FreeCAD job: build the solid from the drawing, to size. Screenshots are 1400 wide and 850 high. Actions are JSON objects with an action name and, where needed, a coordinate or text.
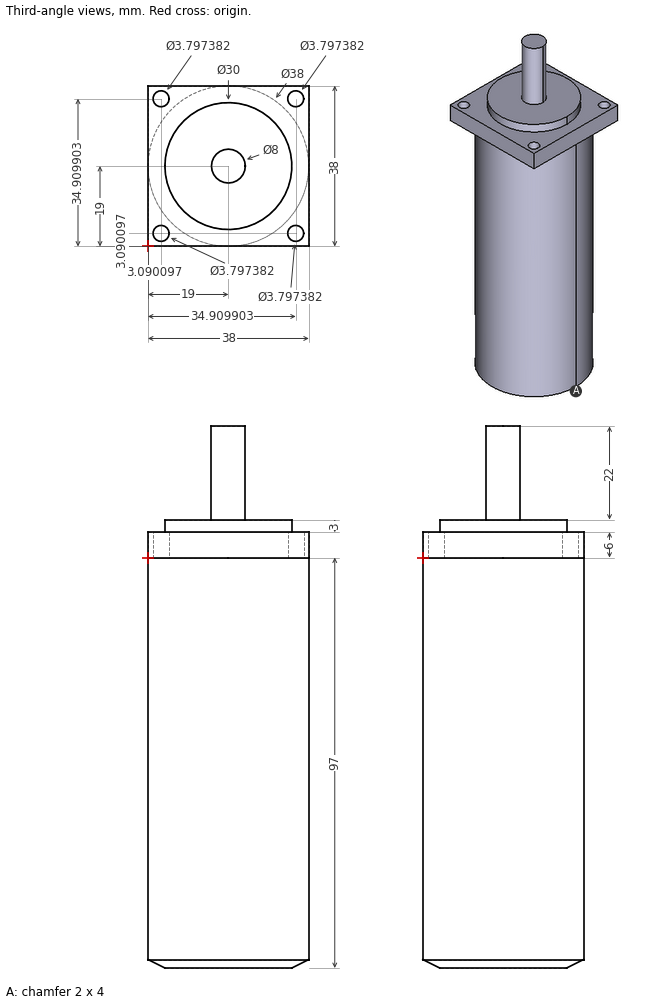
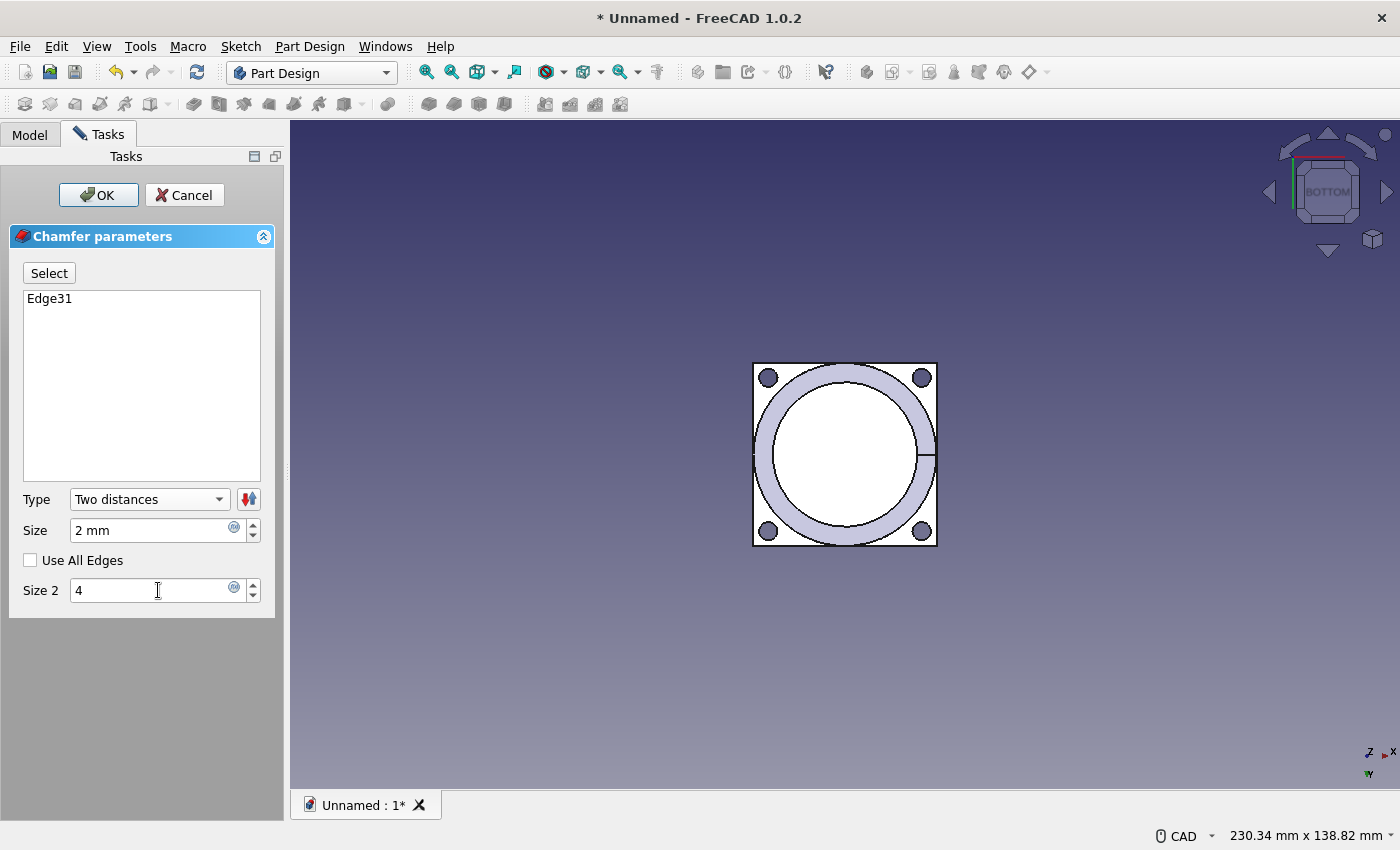
{"action": "left_click", "coordinate": [99, 195]}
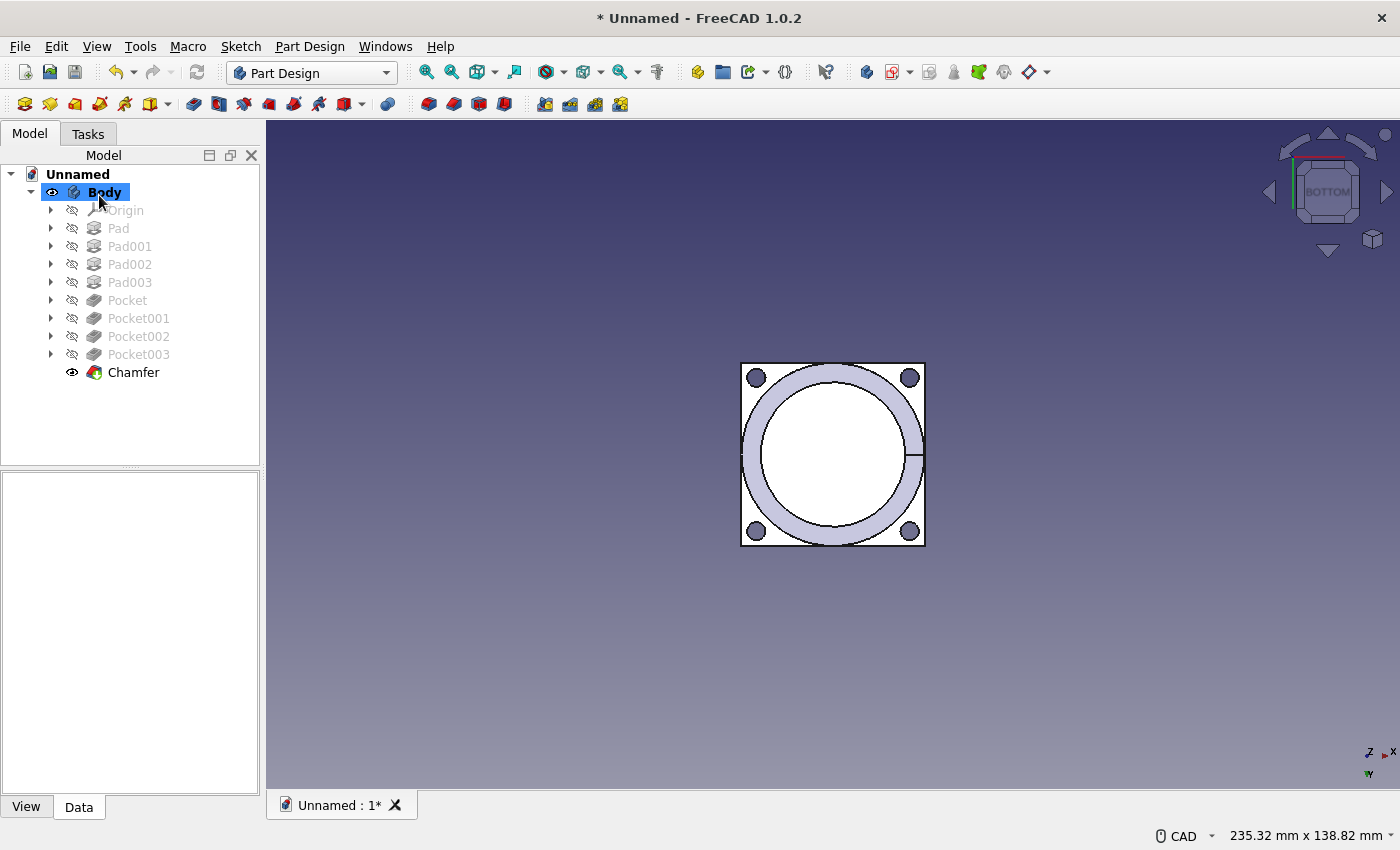
{"action": "key", "text": "0"}